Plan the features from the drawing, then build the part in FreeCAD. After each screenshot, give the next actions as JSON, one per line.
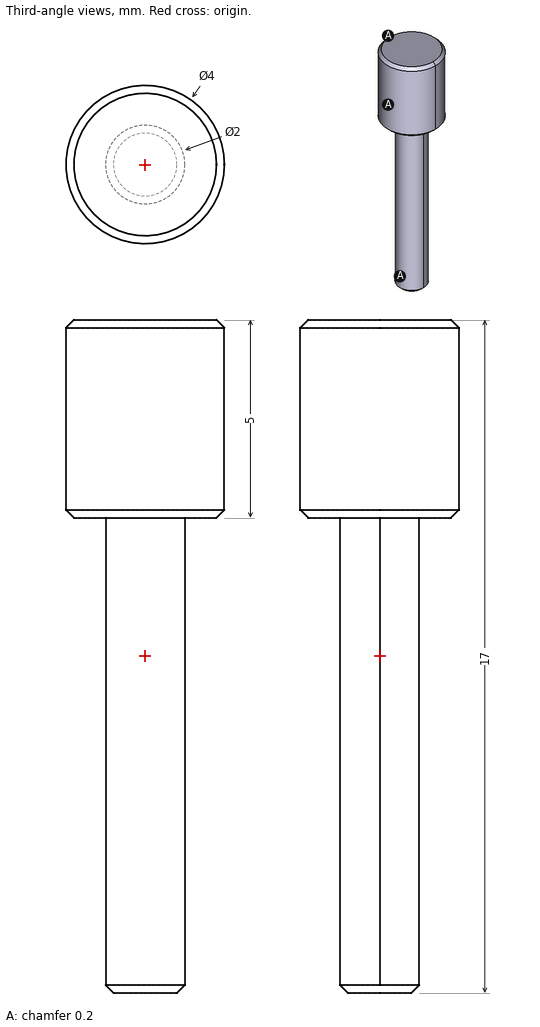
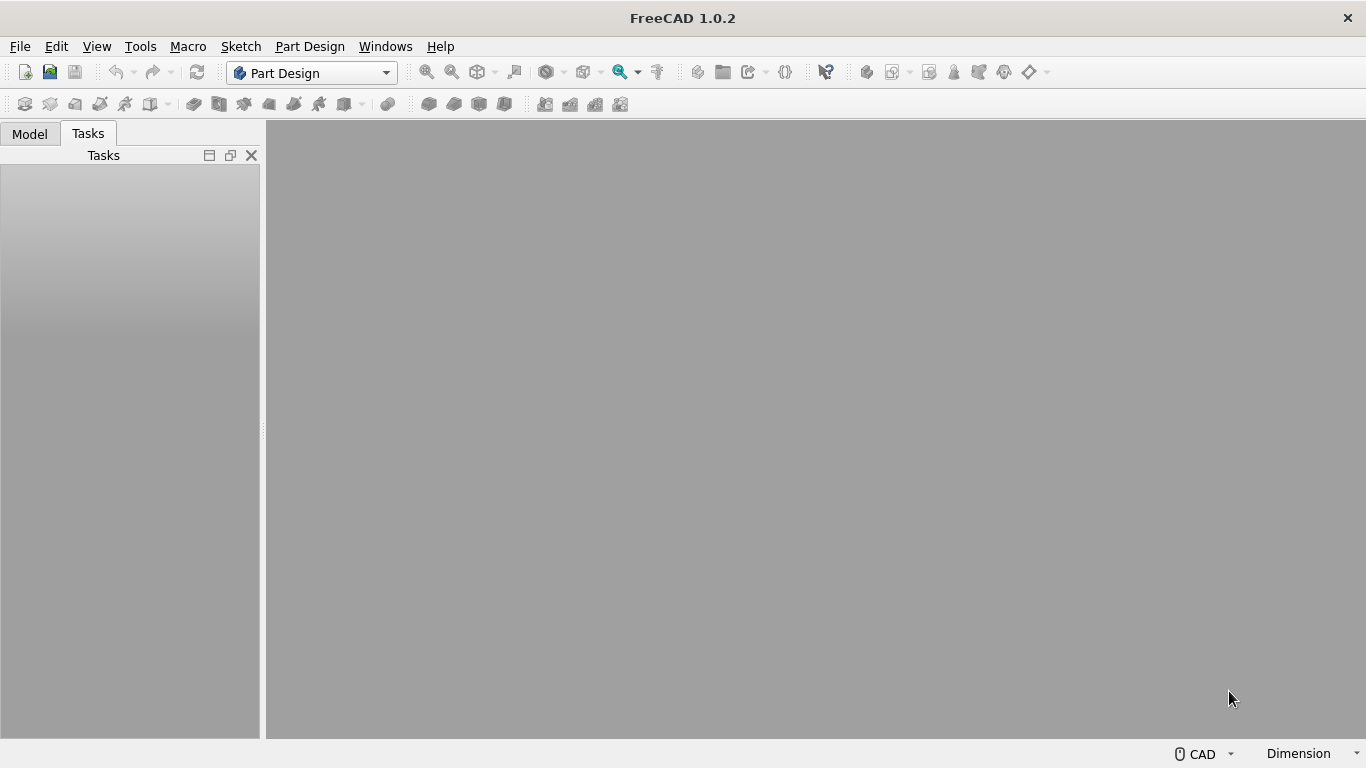
{"action": "left_click", "coordinate": [25, 72]}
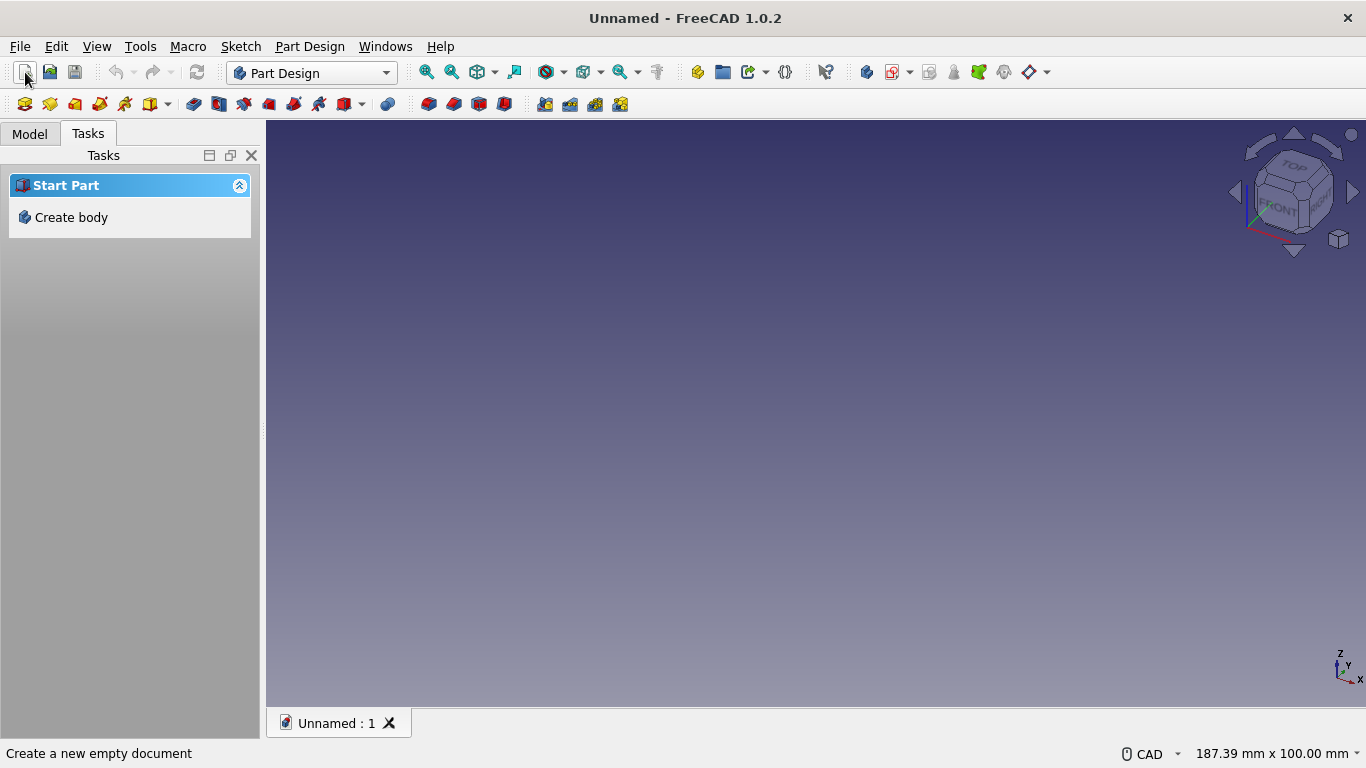
{"action": "left_click", "coordinate": [892, 72]}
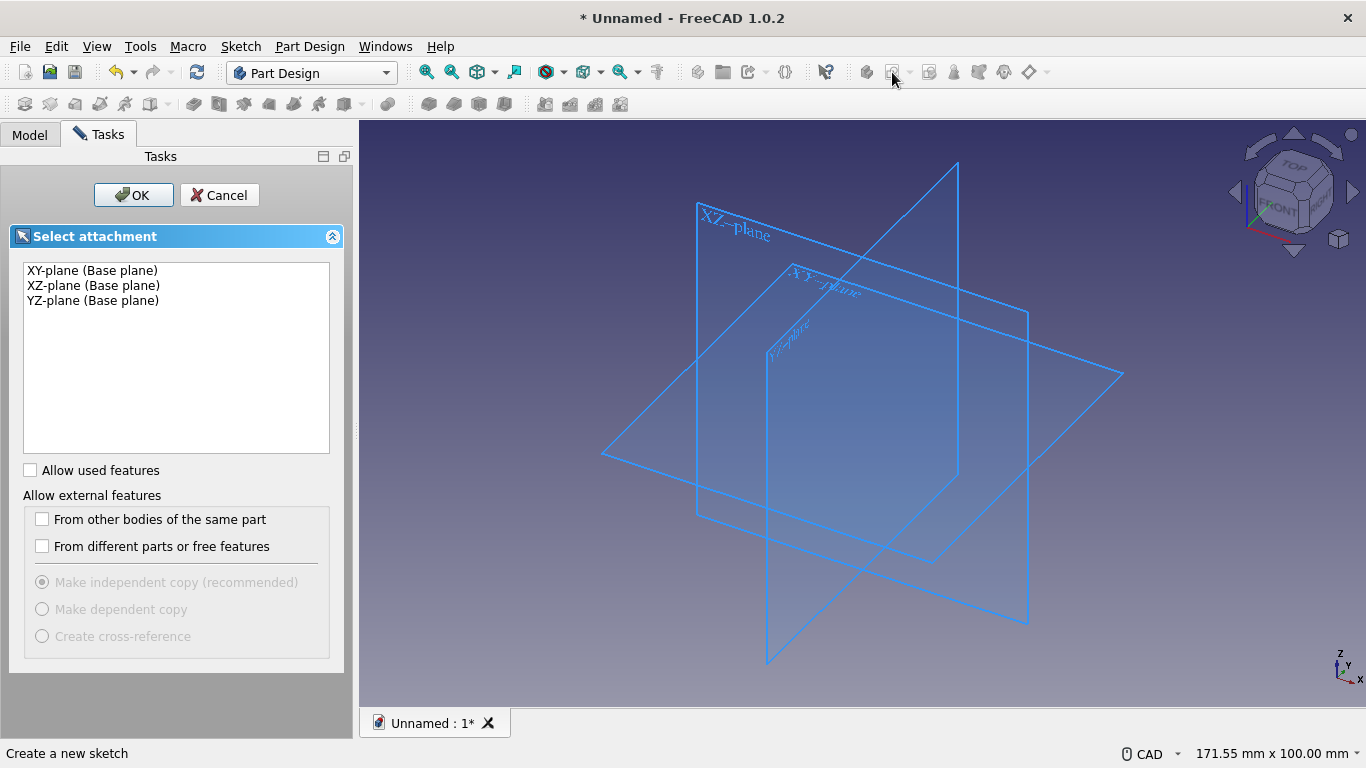
{"action": "left_click", "coordinate": [84, 270]}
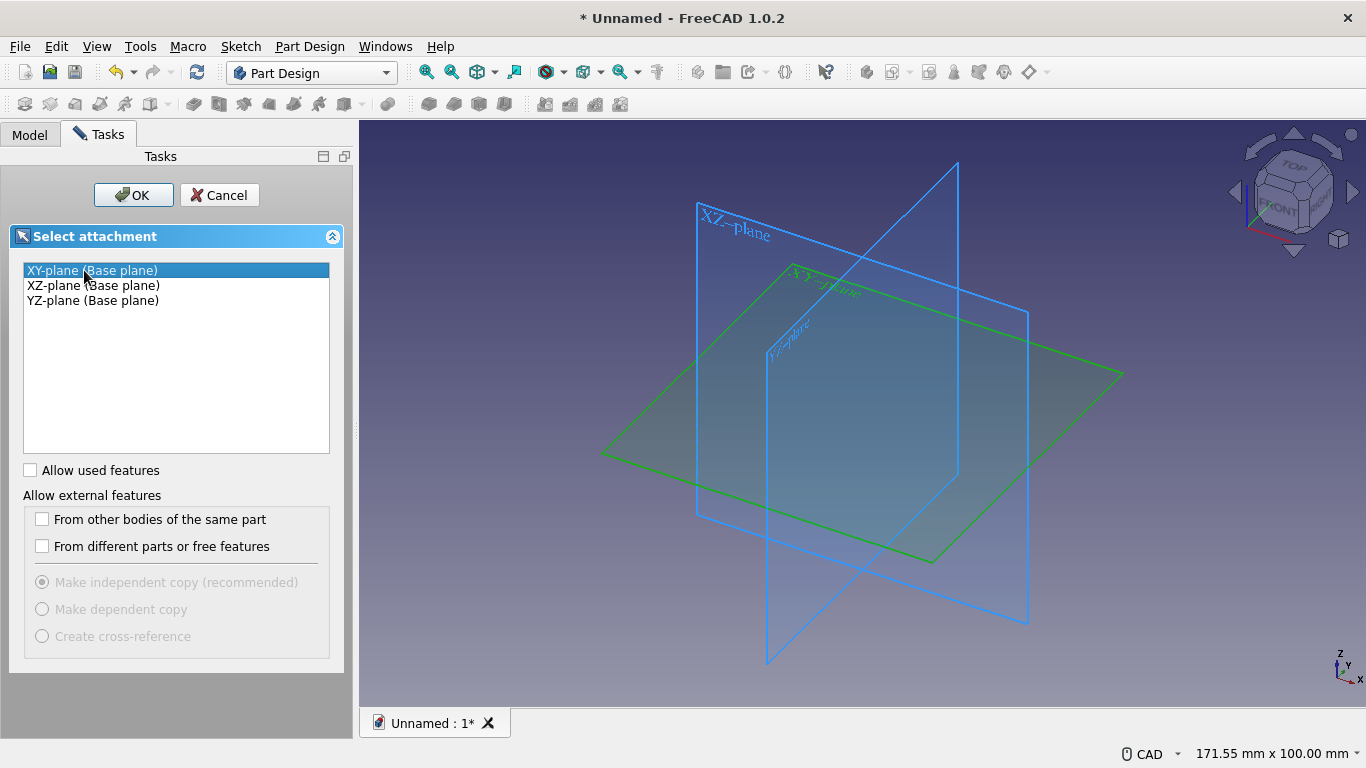
{"action": "left_click", "coordinate": [134, 195]}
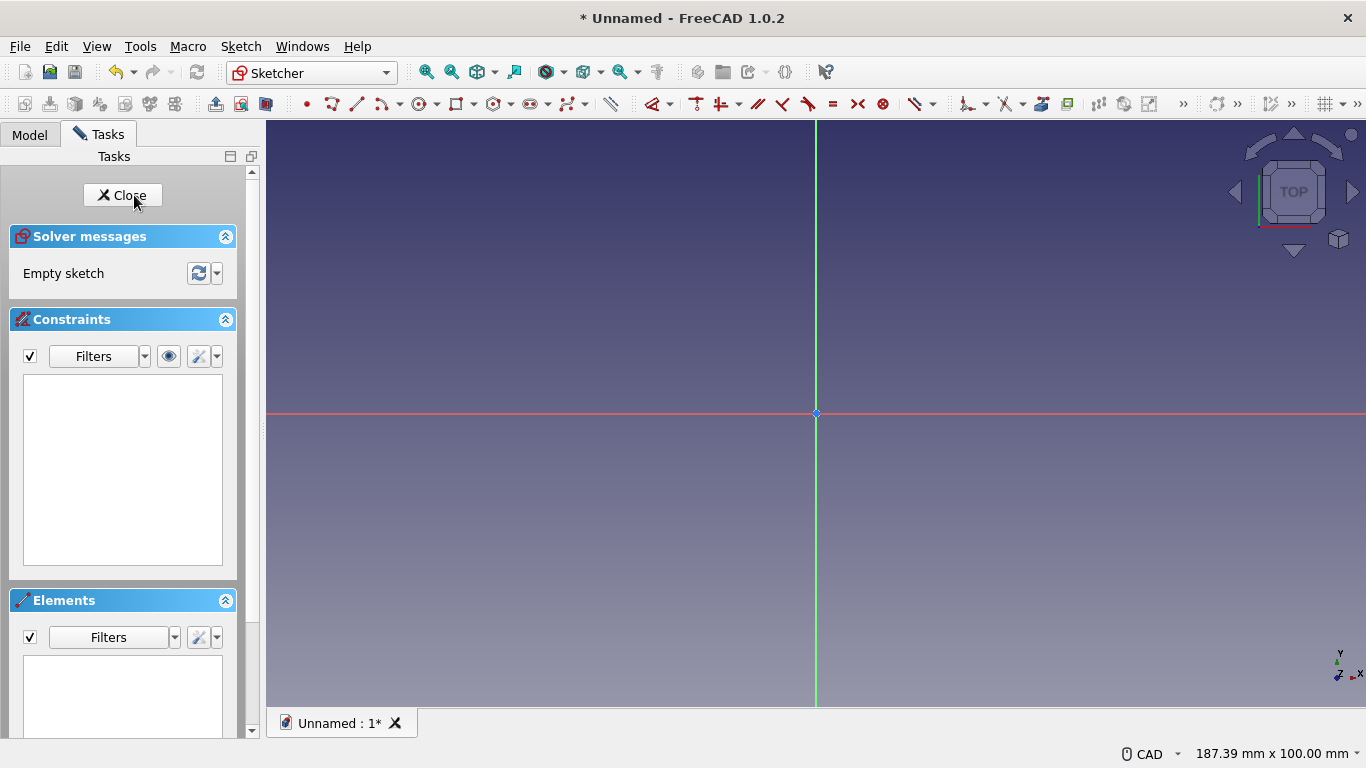
{"action": "scroll", "coordinate": [820, 414], "scroll_direction": "up", "scroll_amount": 15}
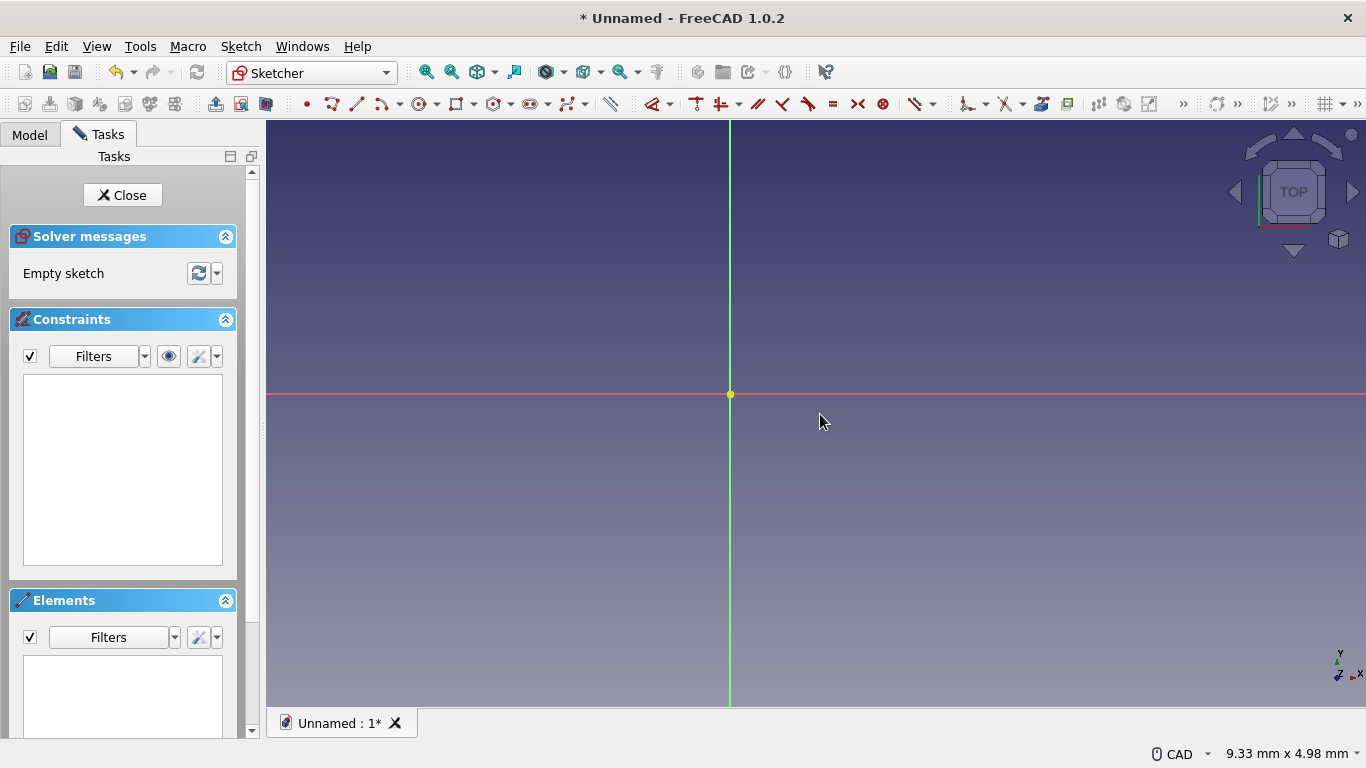
{"action": "scroll", "coordinate": [695, 356], "scroll_direction": "up", "scroll_amount": 2}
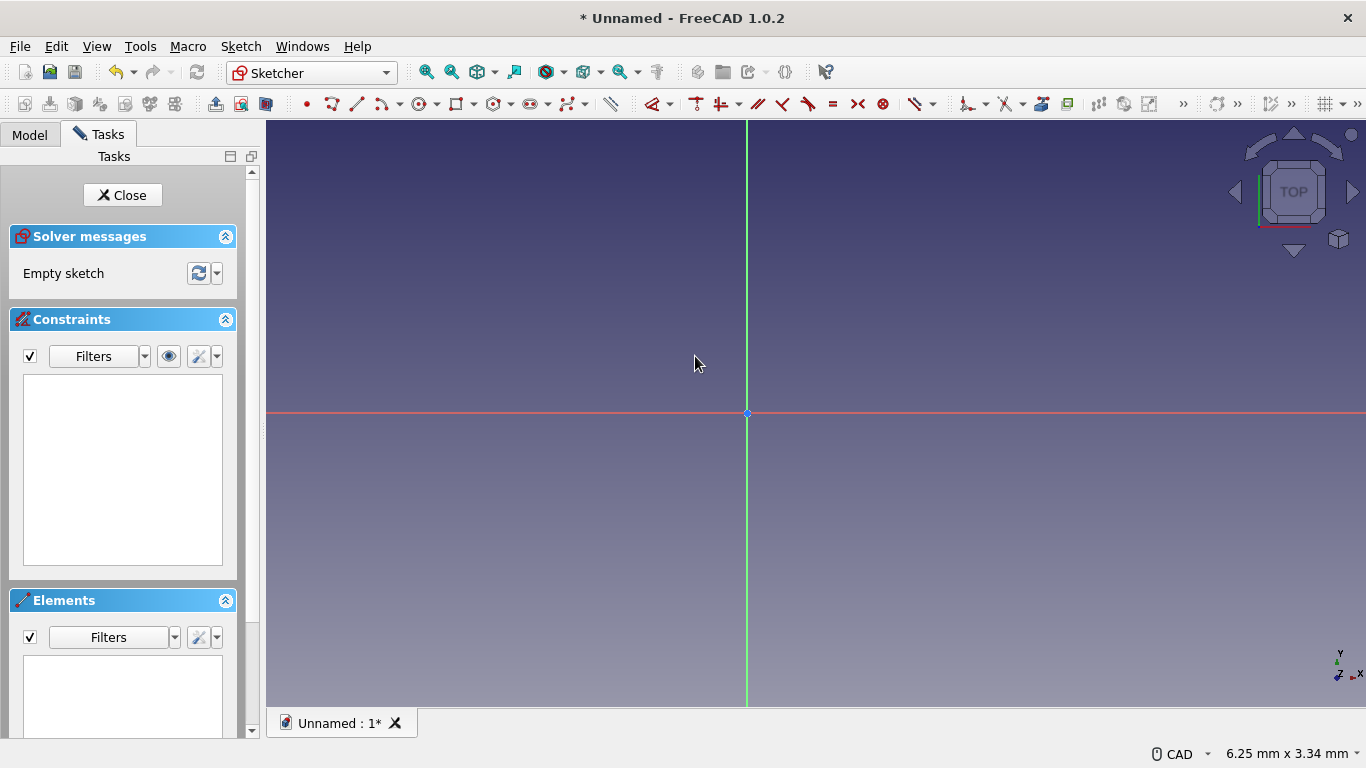
{"action": "left_click", "coordinate": [418, 104]}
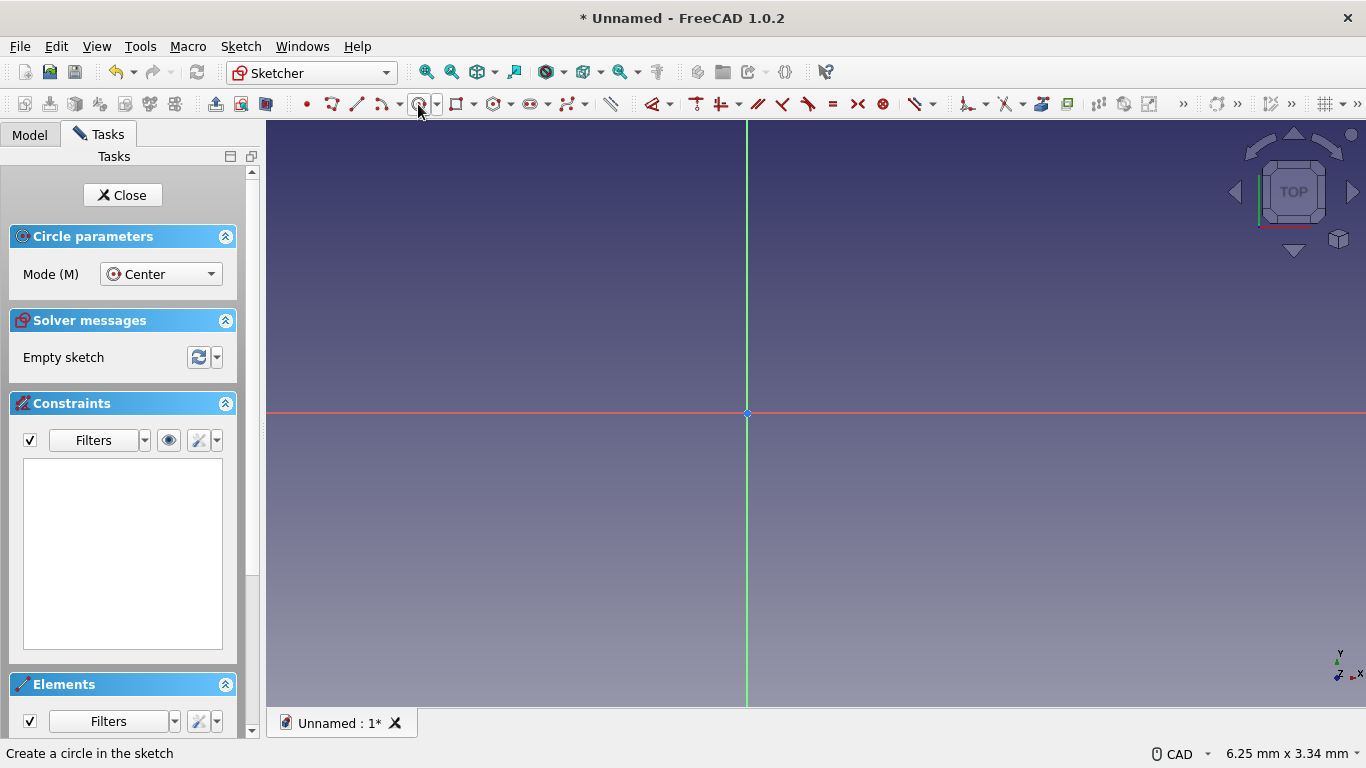
{"action": "left_click", "coordinate": [747, 413]}
{"action": "left_click", "coordinate": [871, 289]}
{"action": "key", "text": "Escape"}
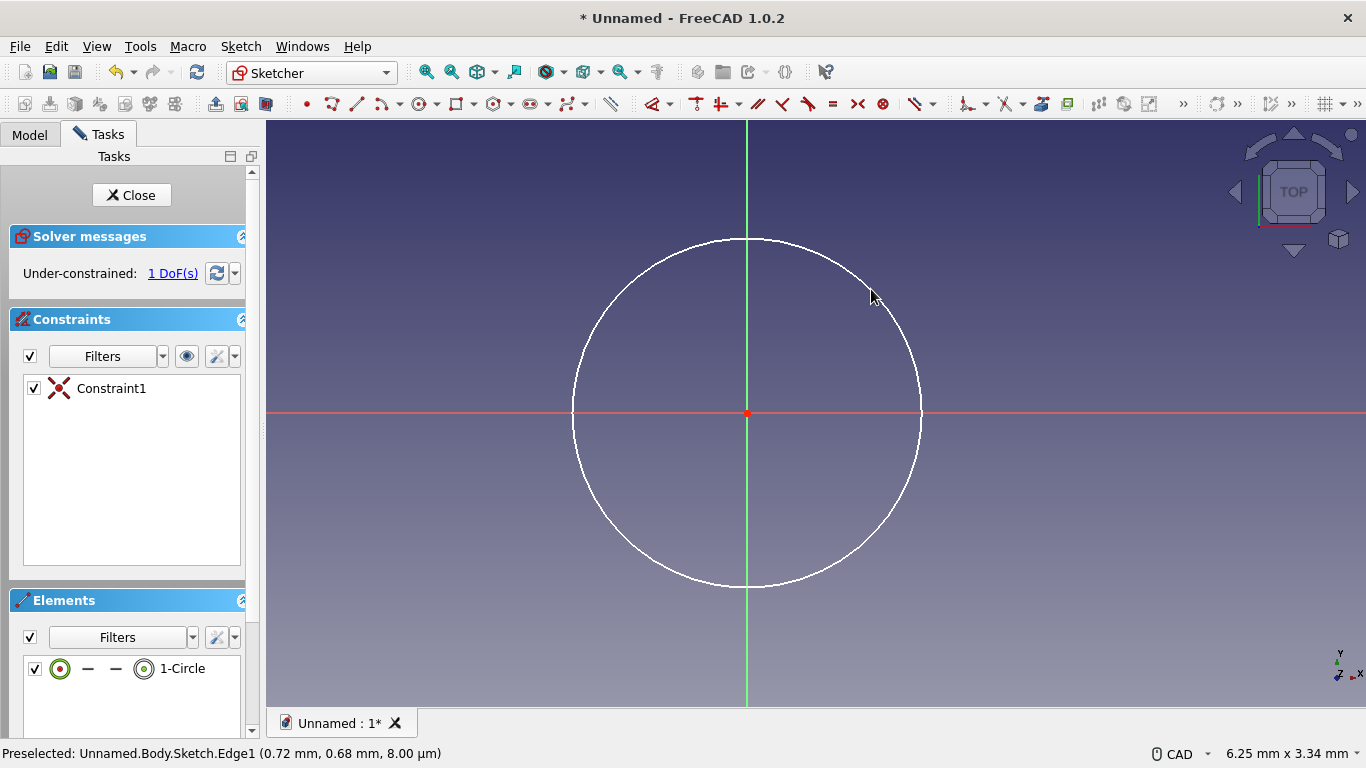
{"action": "left_click", "coordinate": [652, 104]}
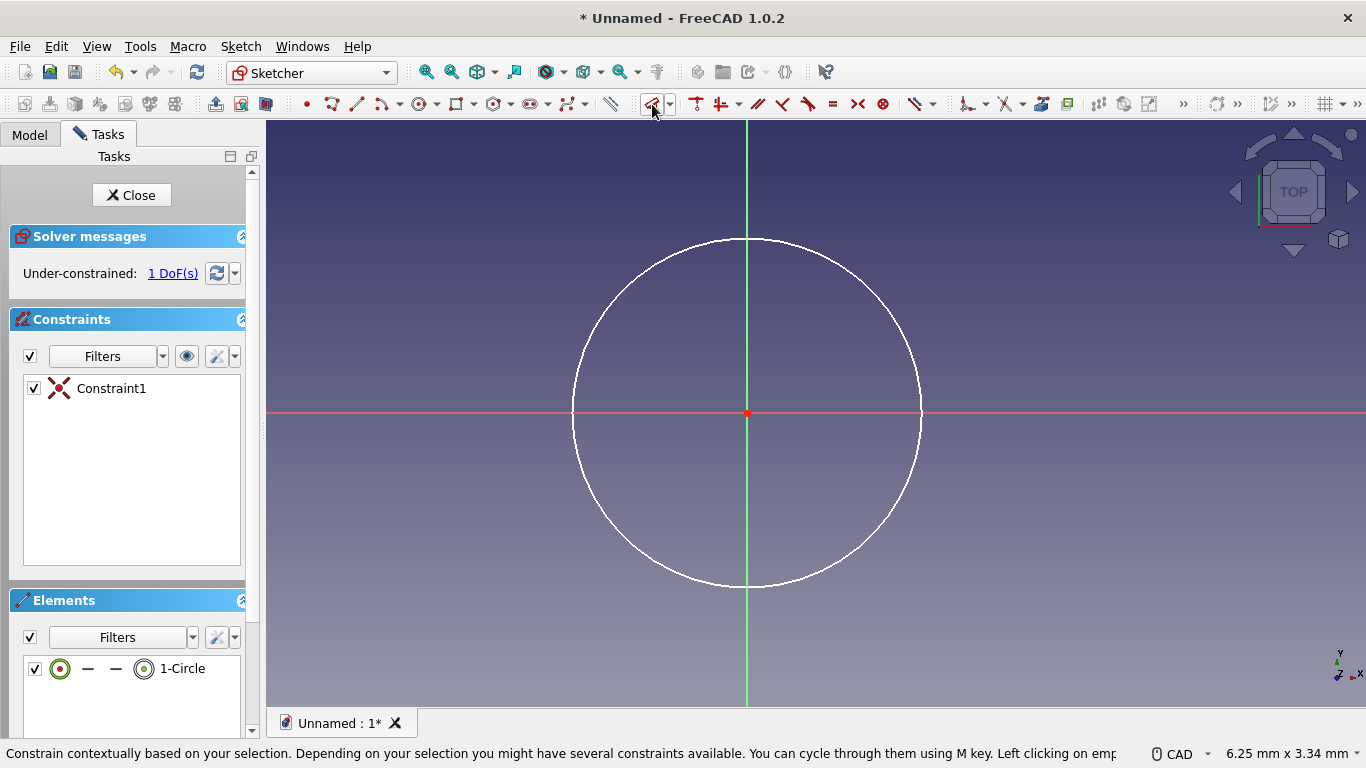
{"action": "left_click", "coordinate": [870, 289]}
{"action": "left_click", "coordinate": [893, 266]}